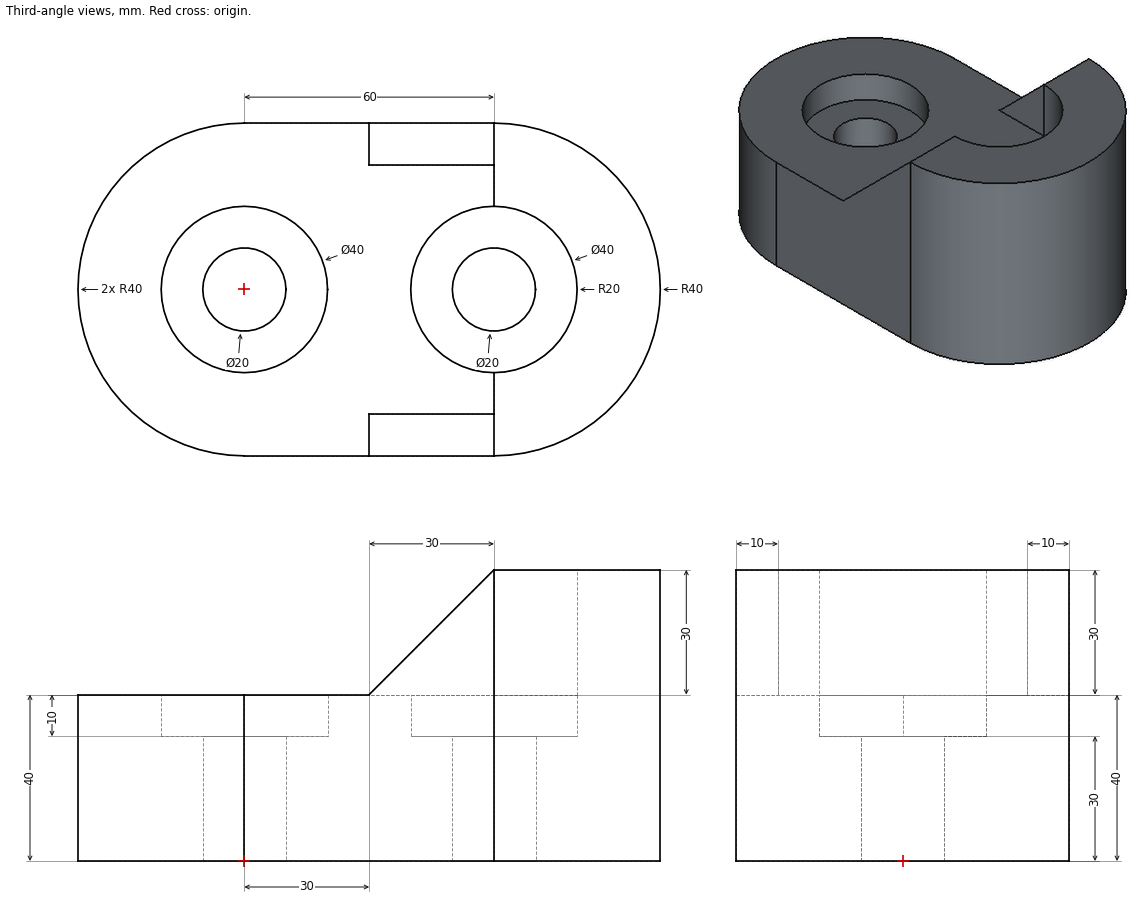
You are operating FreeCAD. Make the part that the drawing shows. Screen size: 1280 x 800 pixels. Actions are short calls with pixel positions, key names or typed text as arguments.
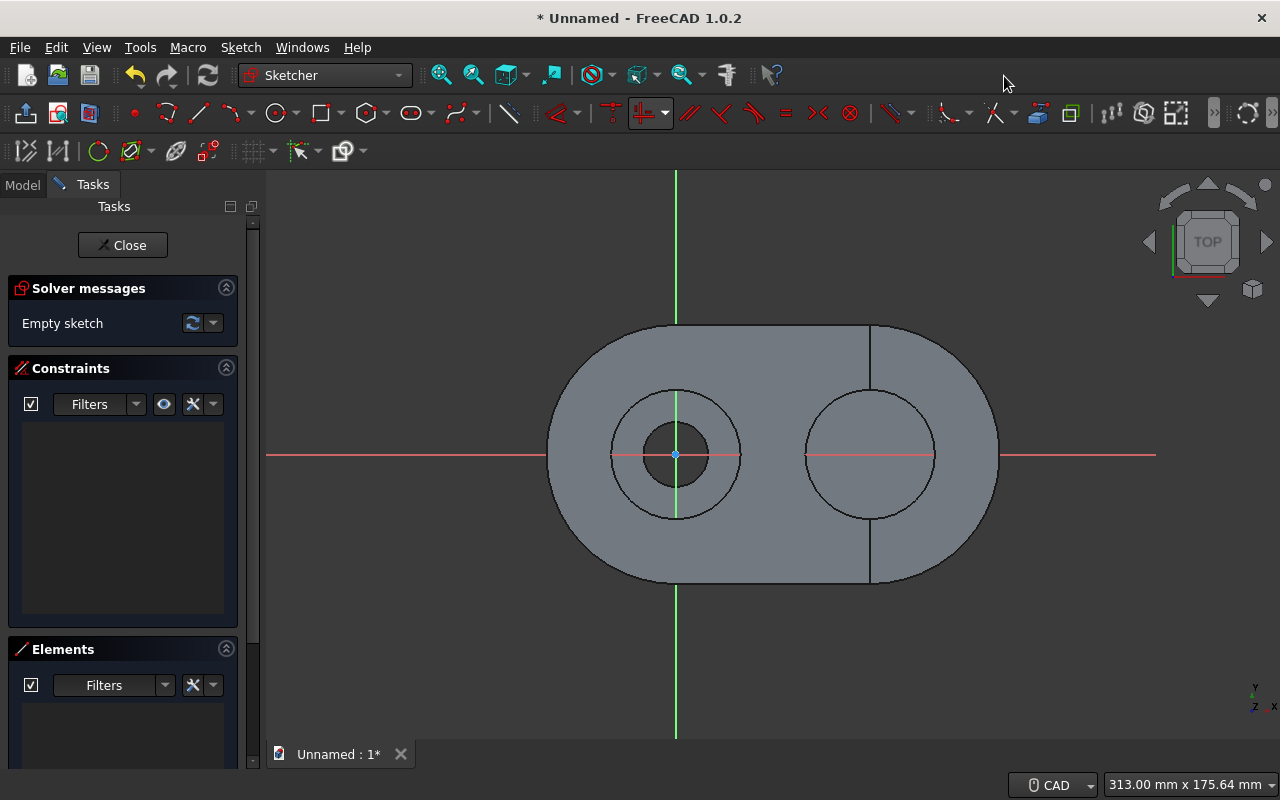
scroll(903, 455, up, 9)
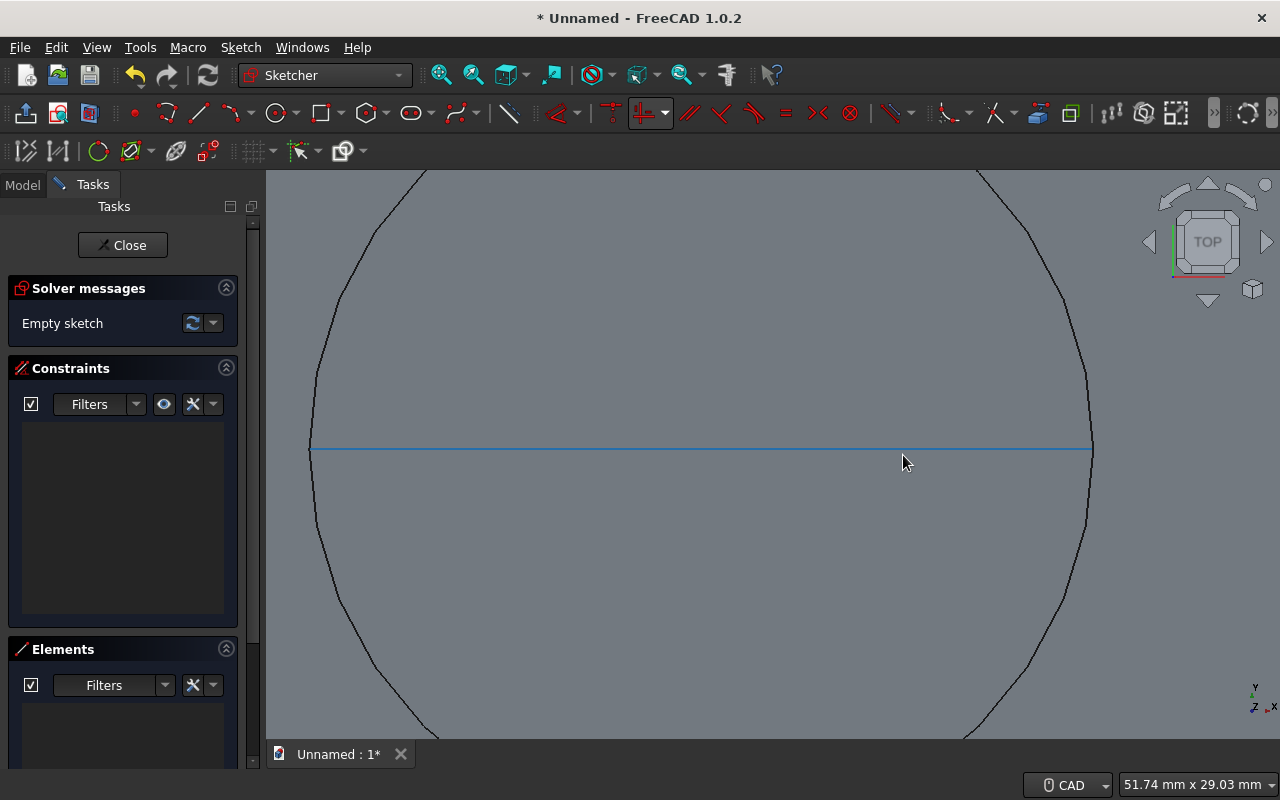
click(276, 114)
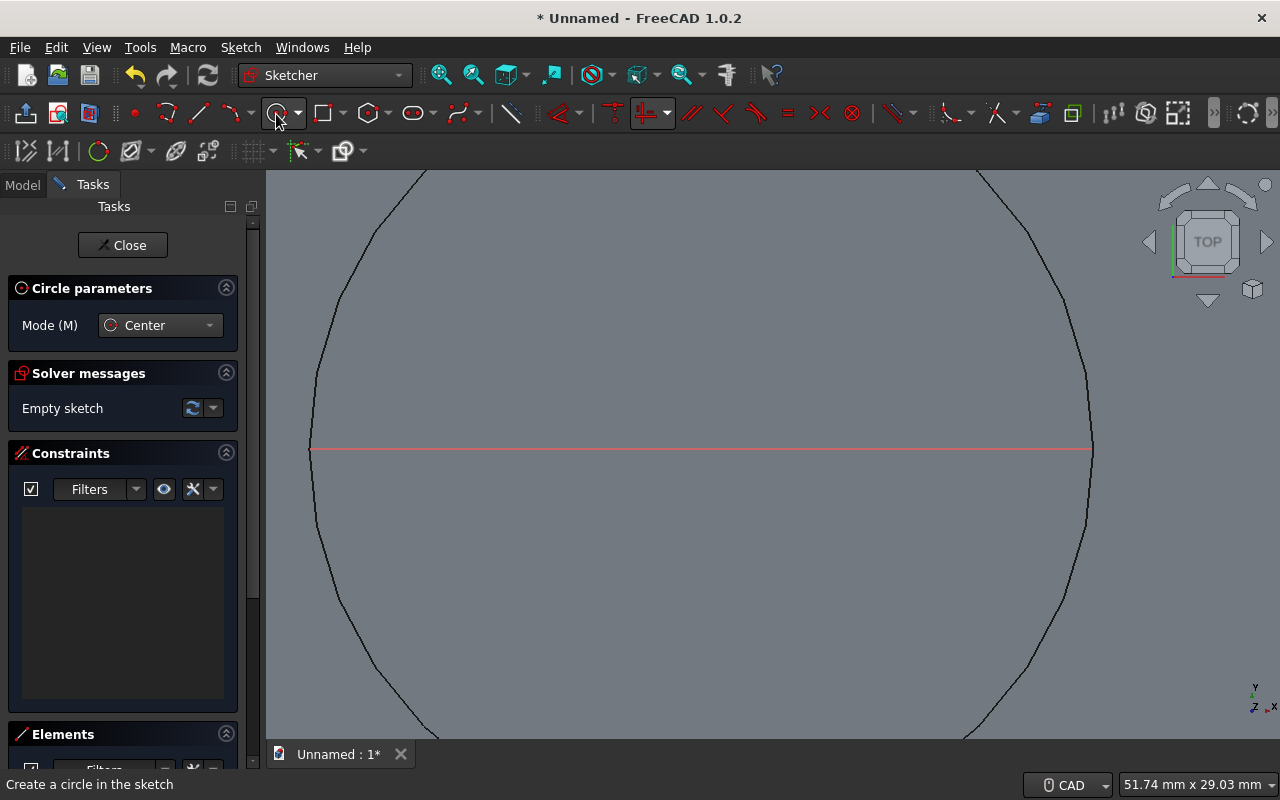
click(701, 449)
move(840, 311)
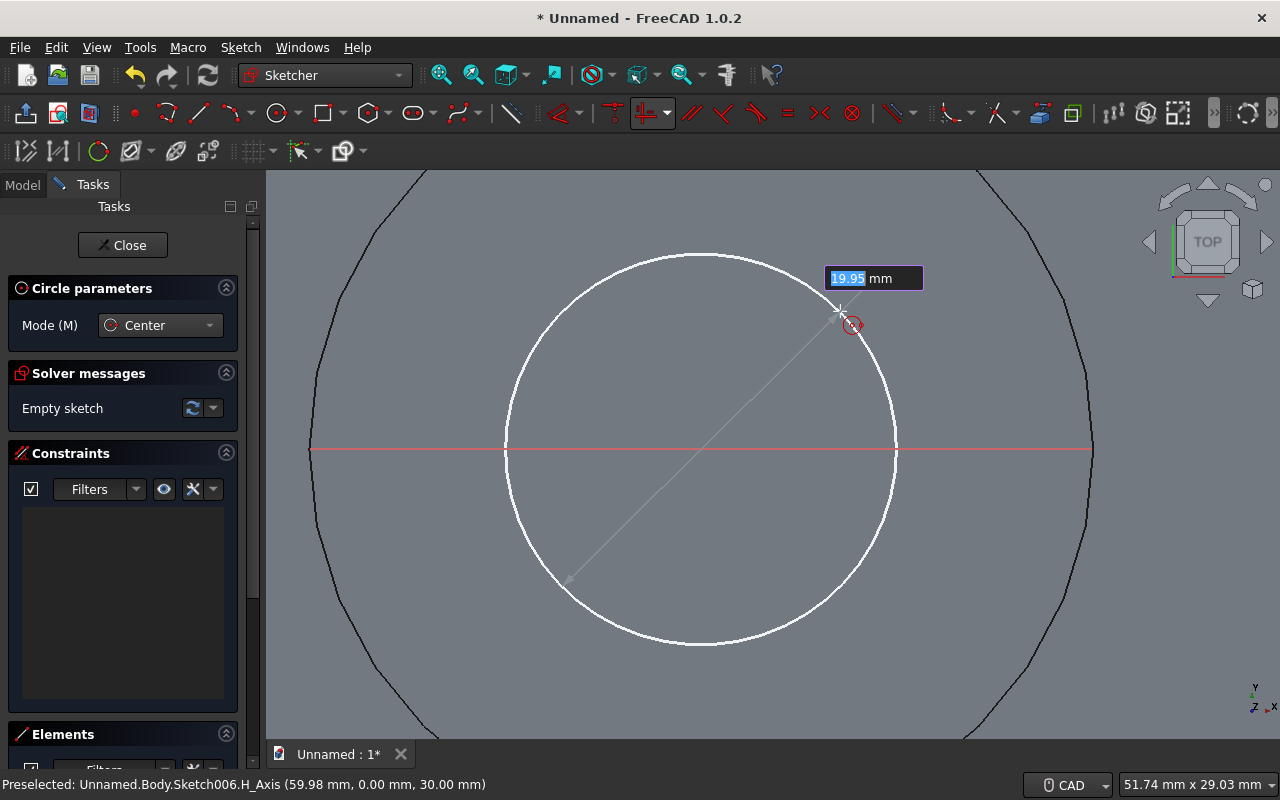
text(20)
key(Return)
key(Escape)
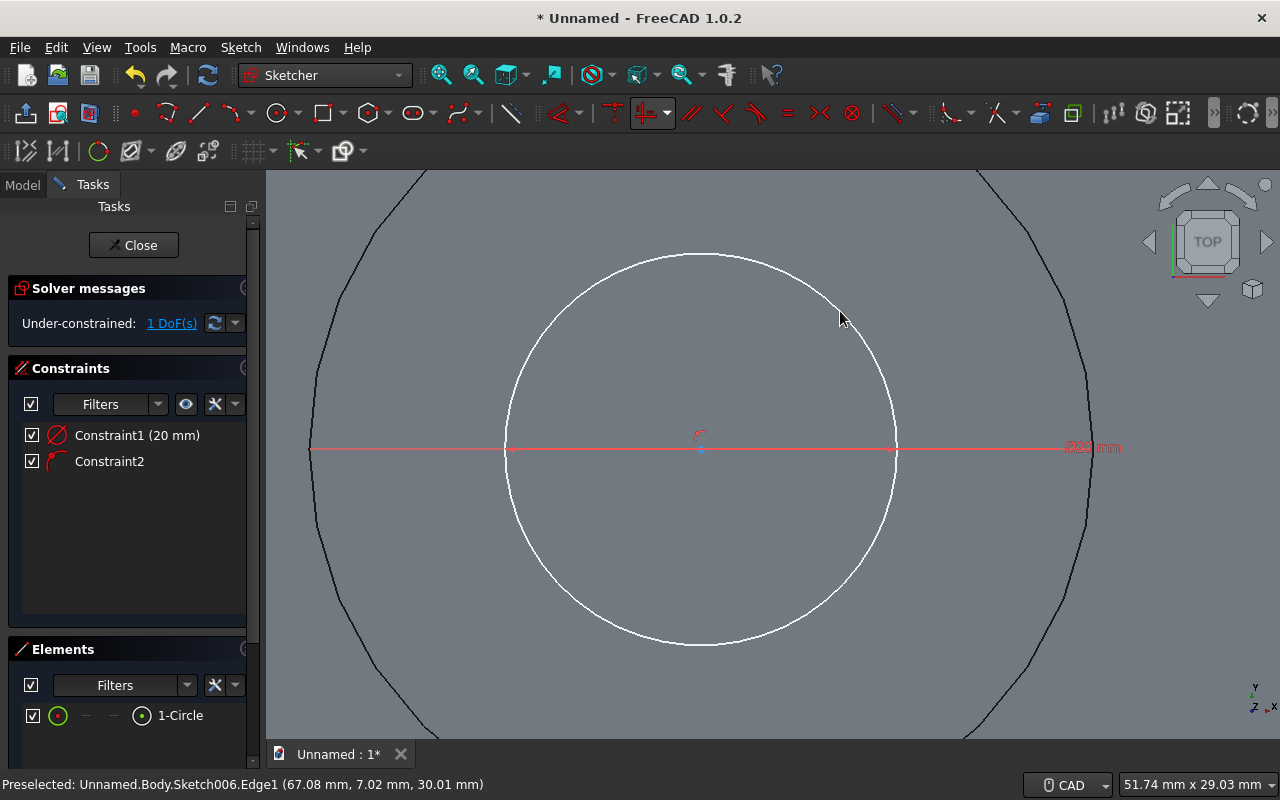
click(558, 114)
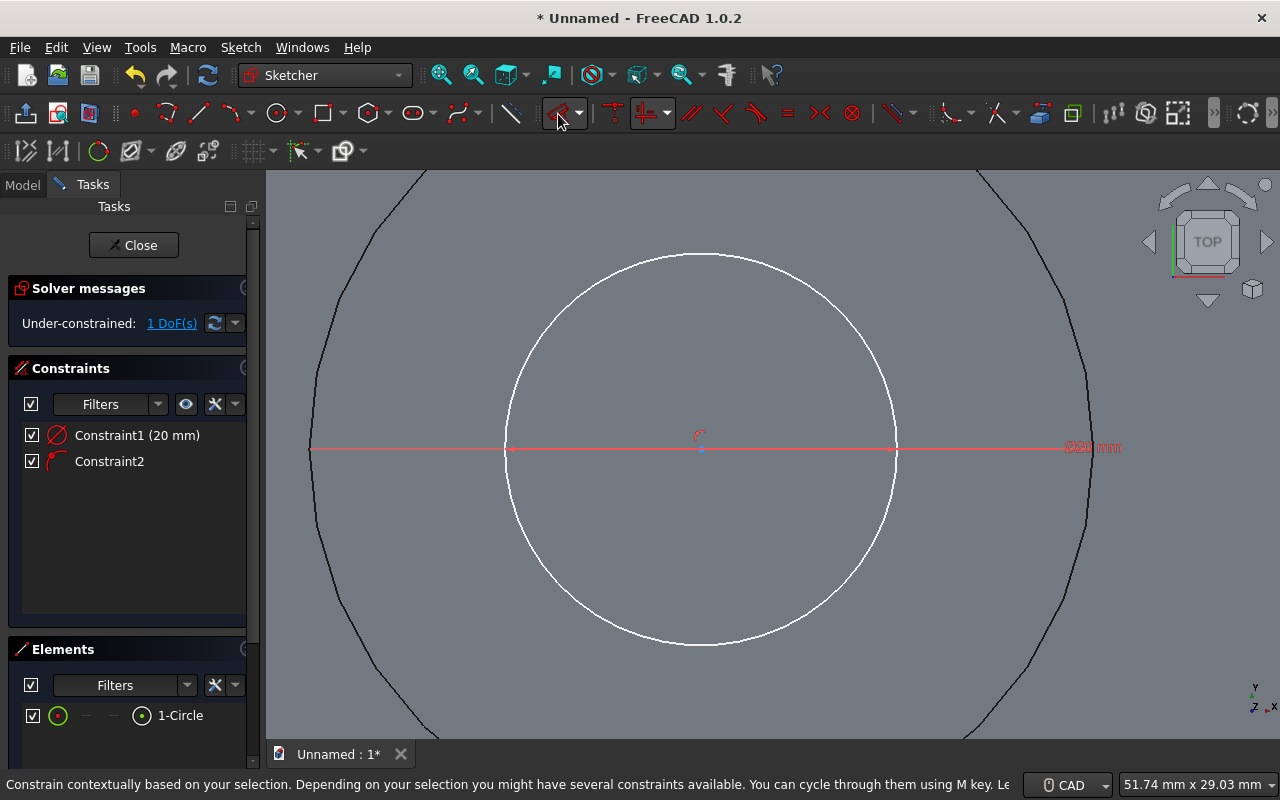
click(701, 449)
click(404, 483)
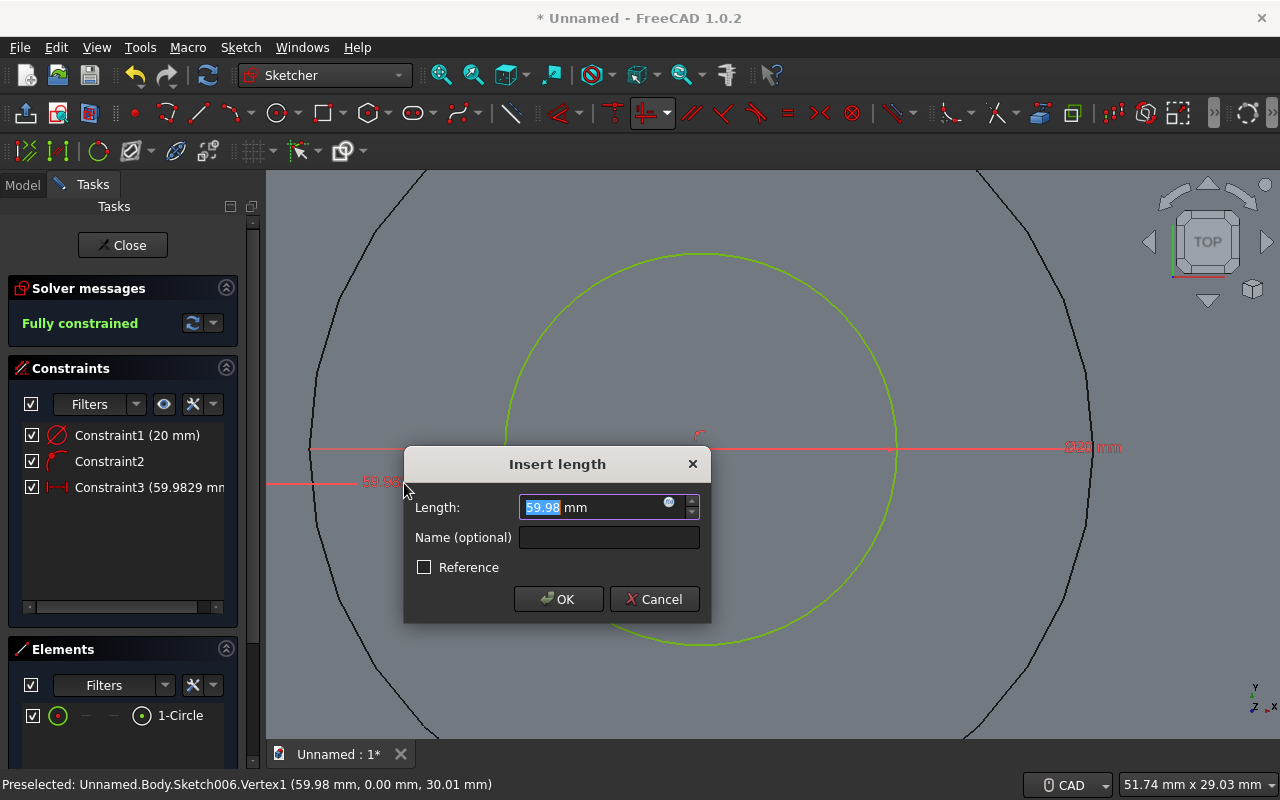
text(60)
key(Return)
key(Escape)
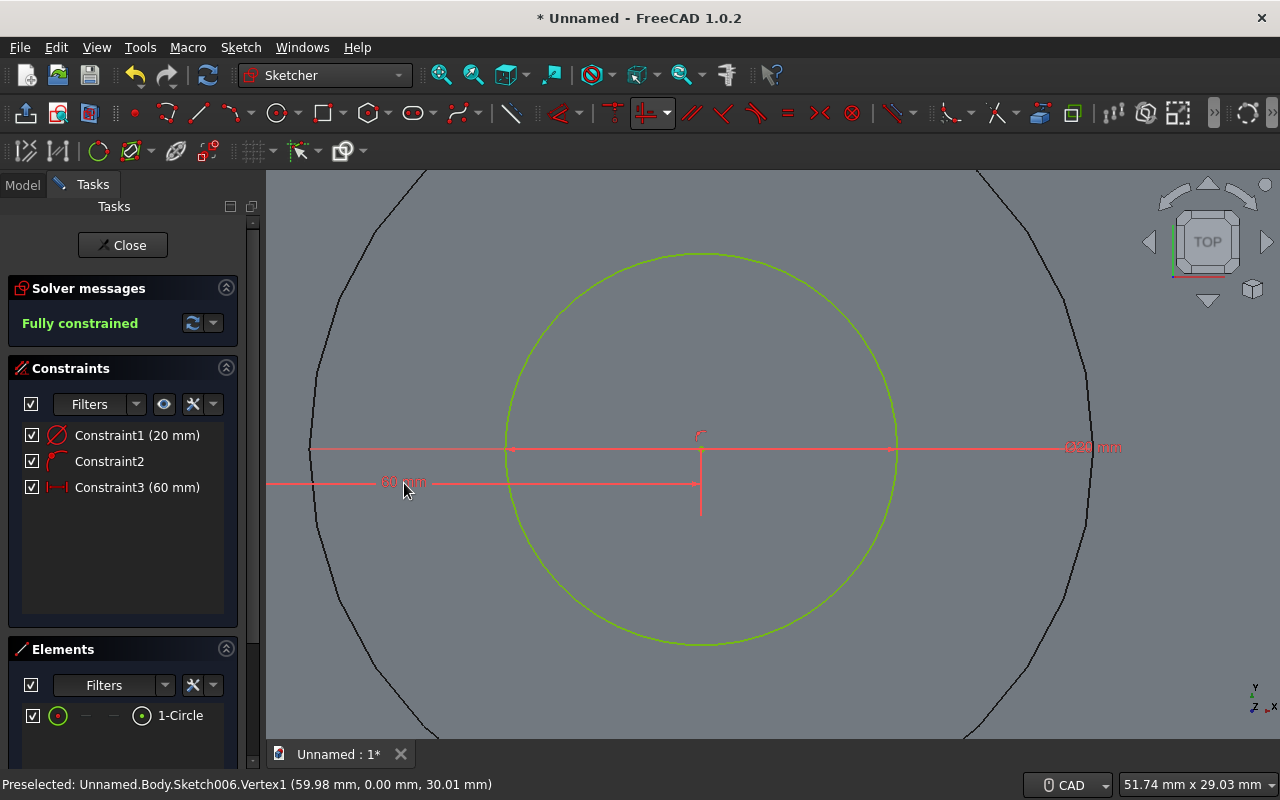
click(123, 245)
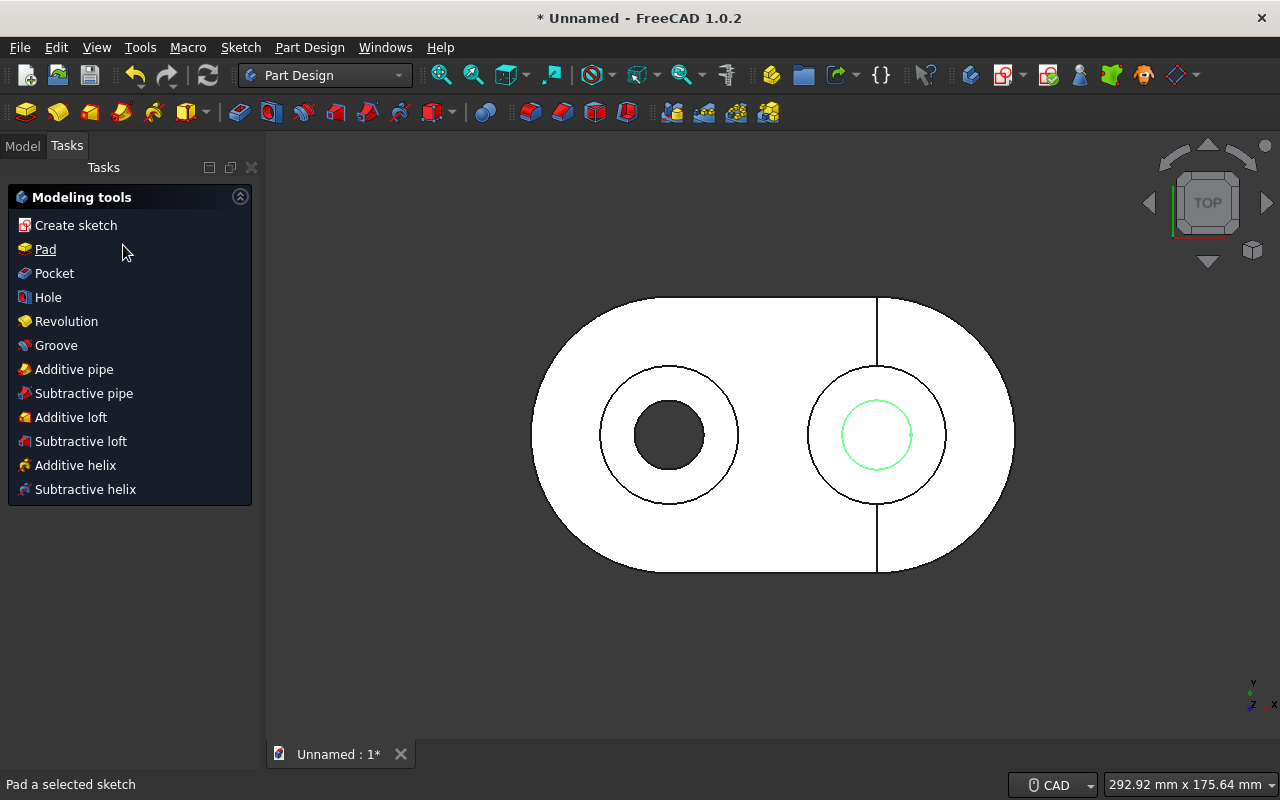
click(240, 112)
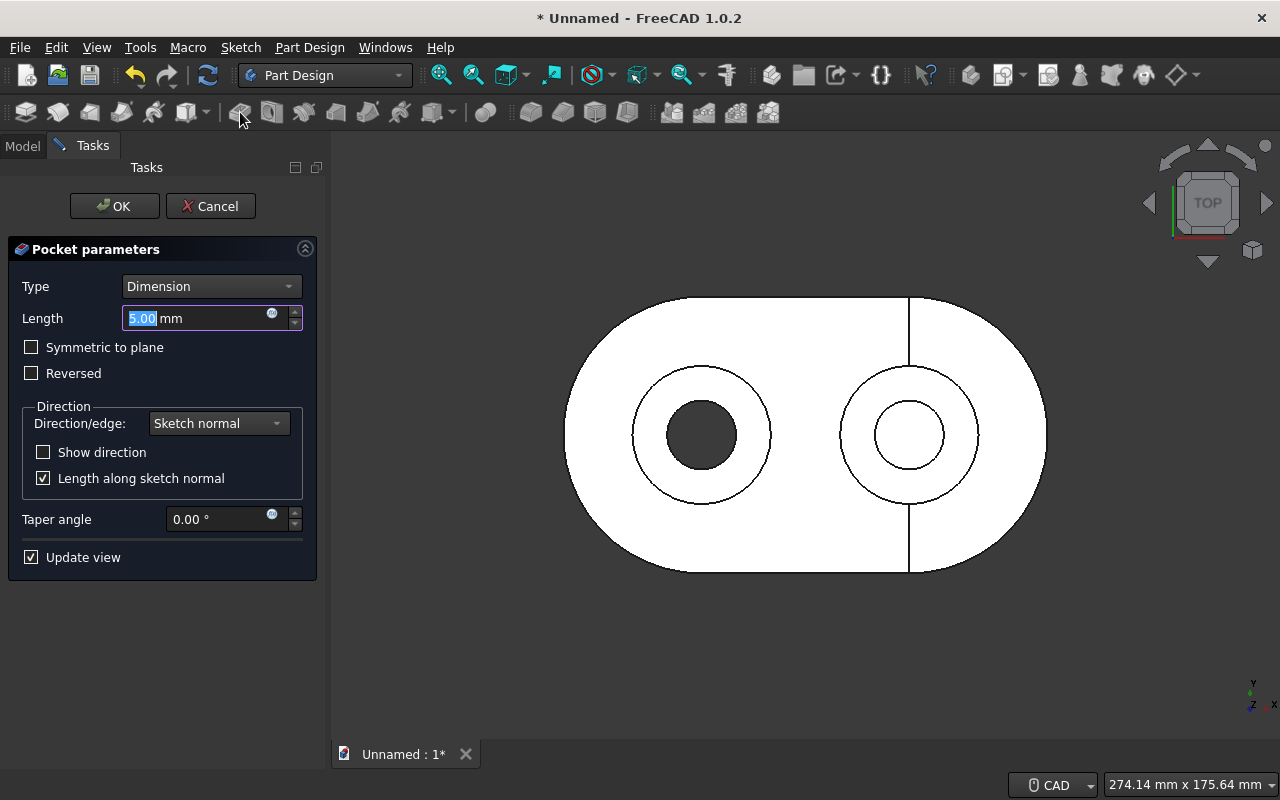
text(30)
key(Tab)